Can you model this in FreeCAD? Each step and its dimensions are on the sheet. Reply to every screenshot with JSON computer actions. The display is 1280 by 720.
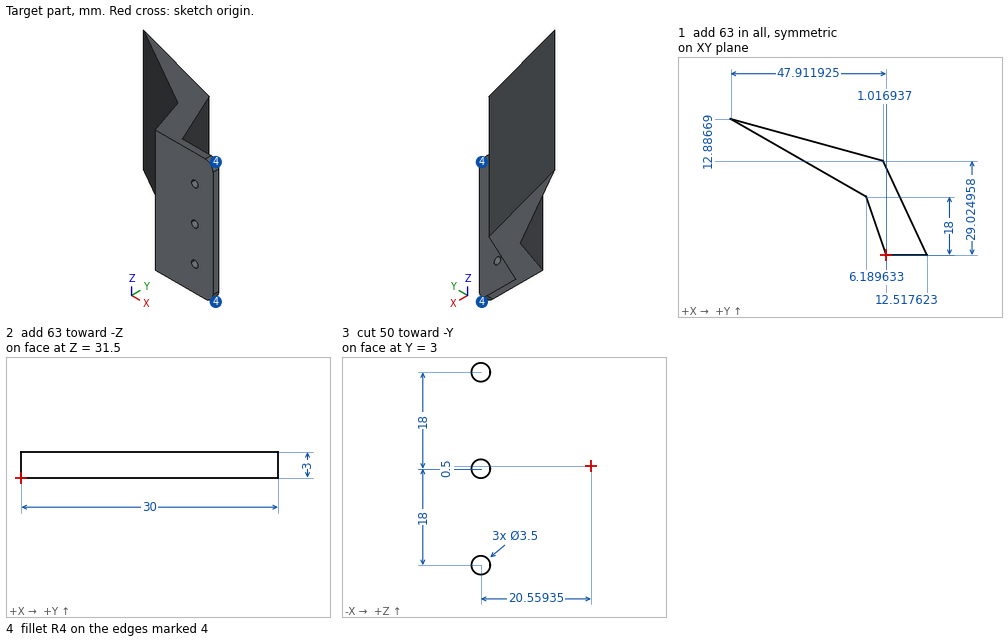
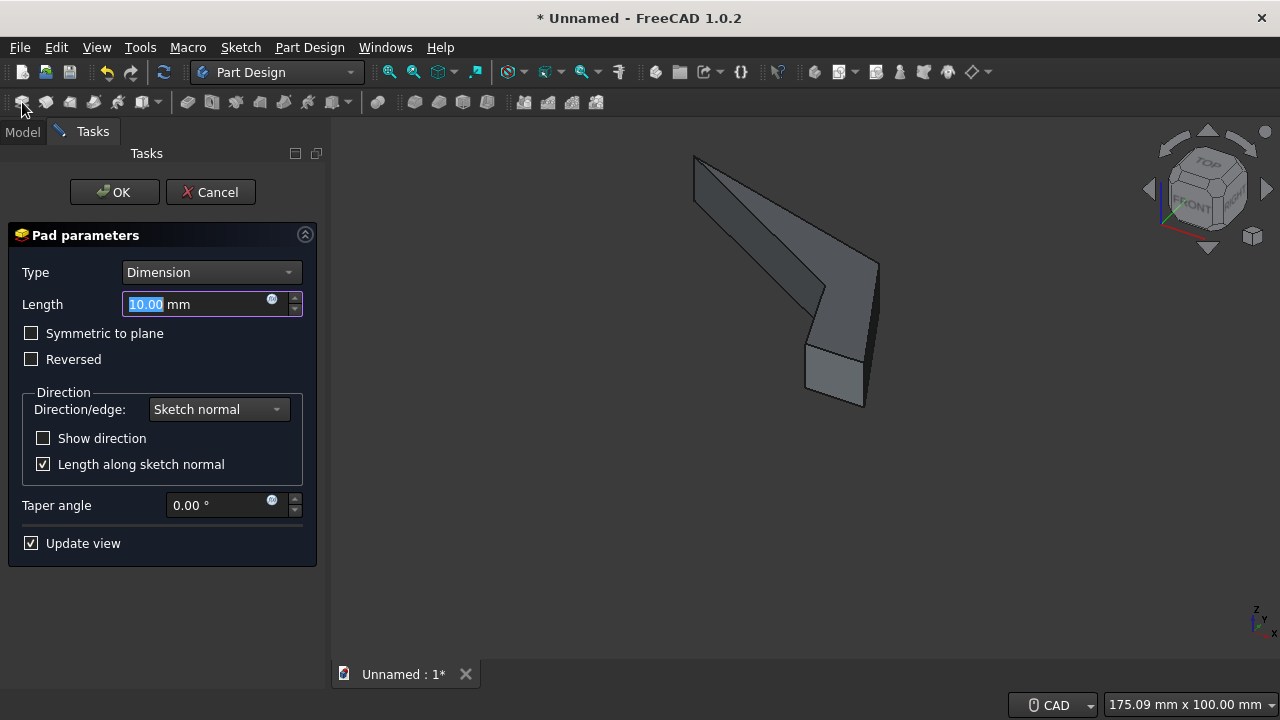
{"action": "type", "text": "63"}
{"action": "key", "text": "Tab"}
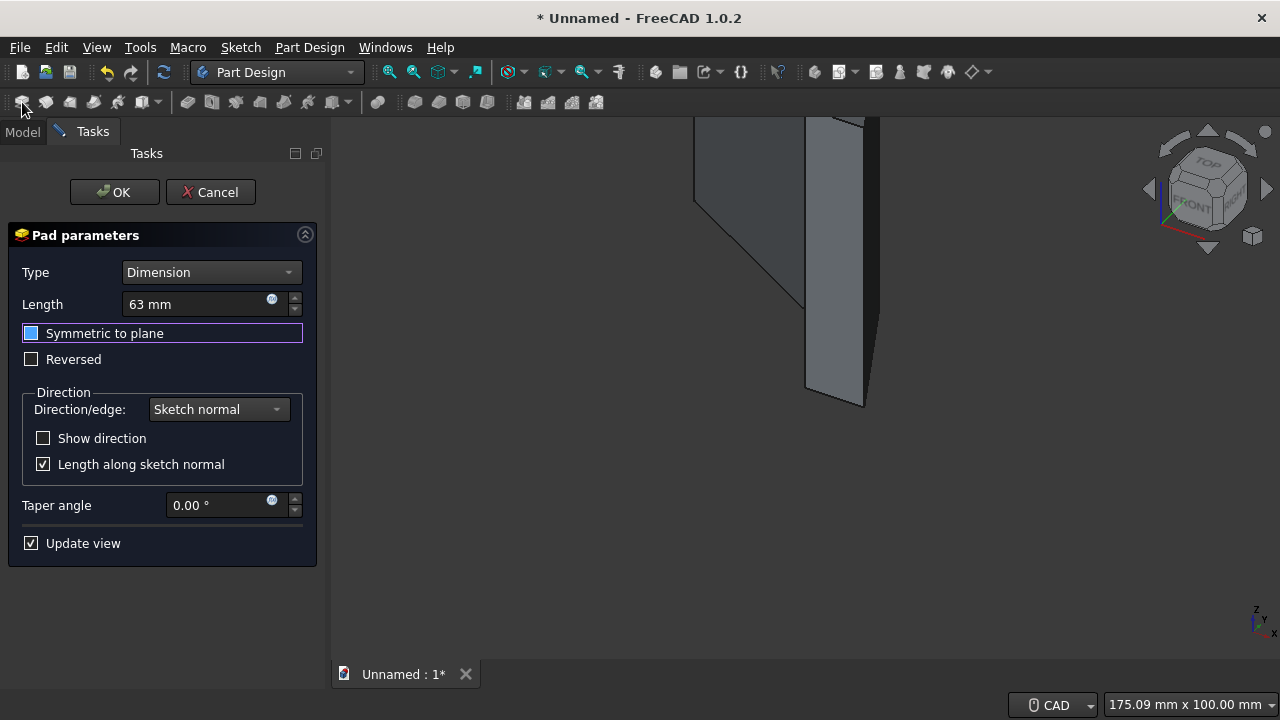
{"action": "left_click", "coordinate": [30, 333]}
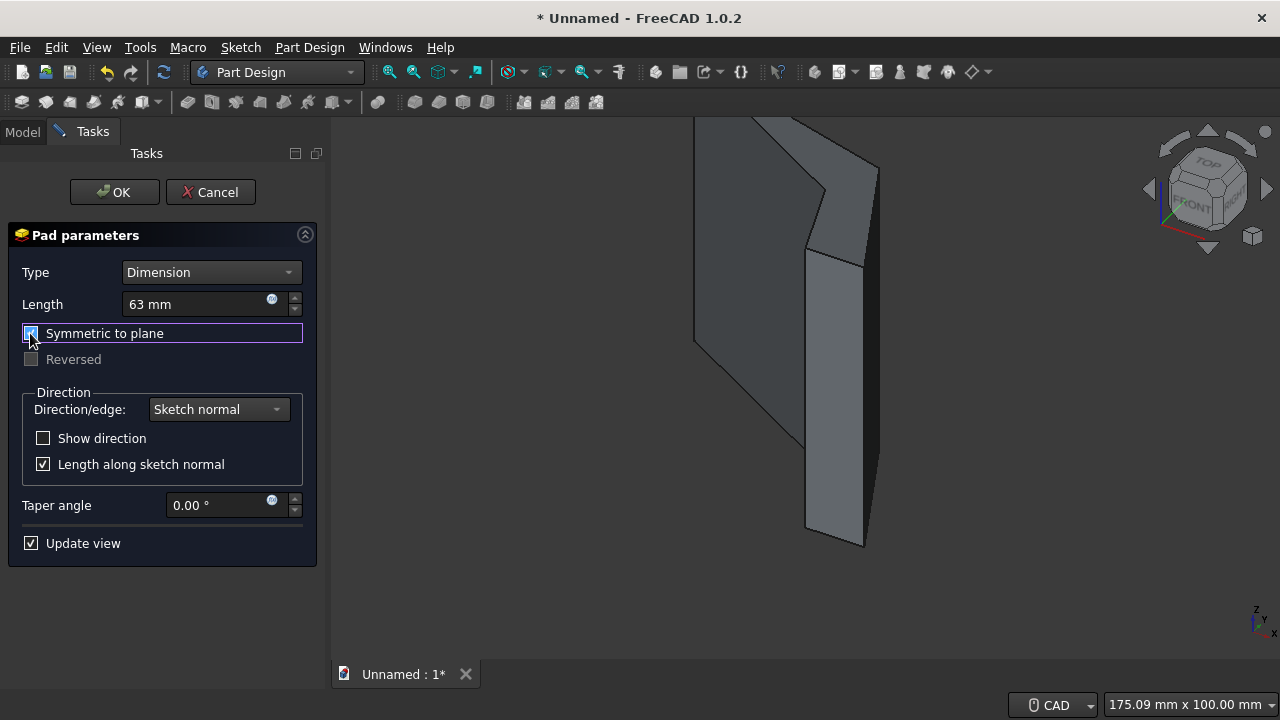
{"action": "left_click", "coordinate": [115, 192]}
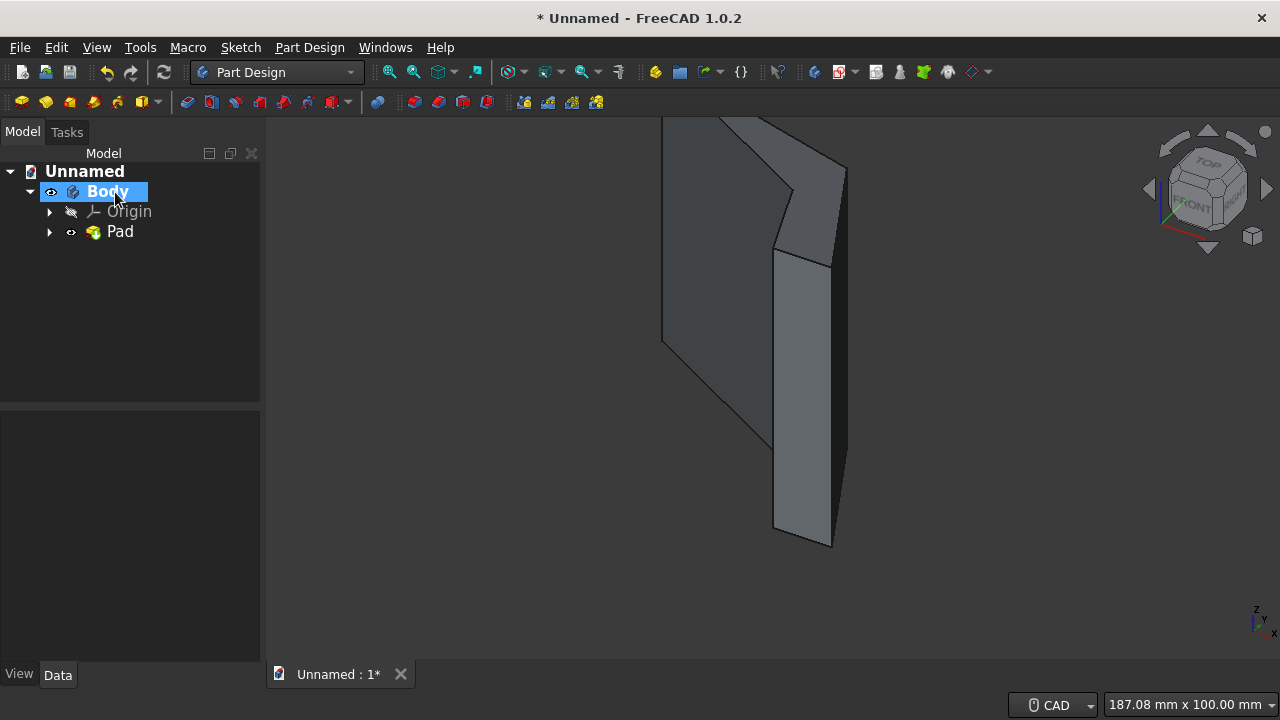
{"action": "key", "text": "v f"}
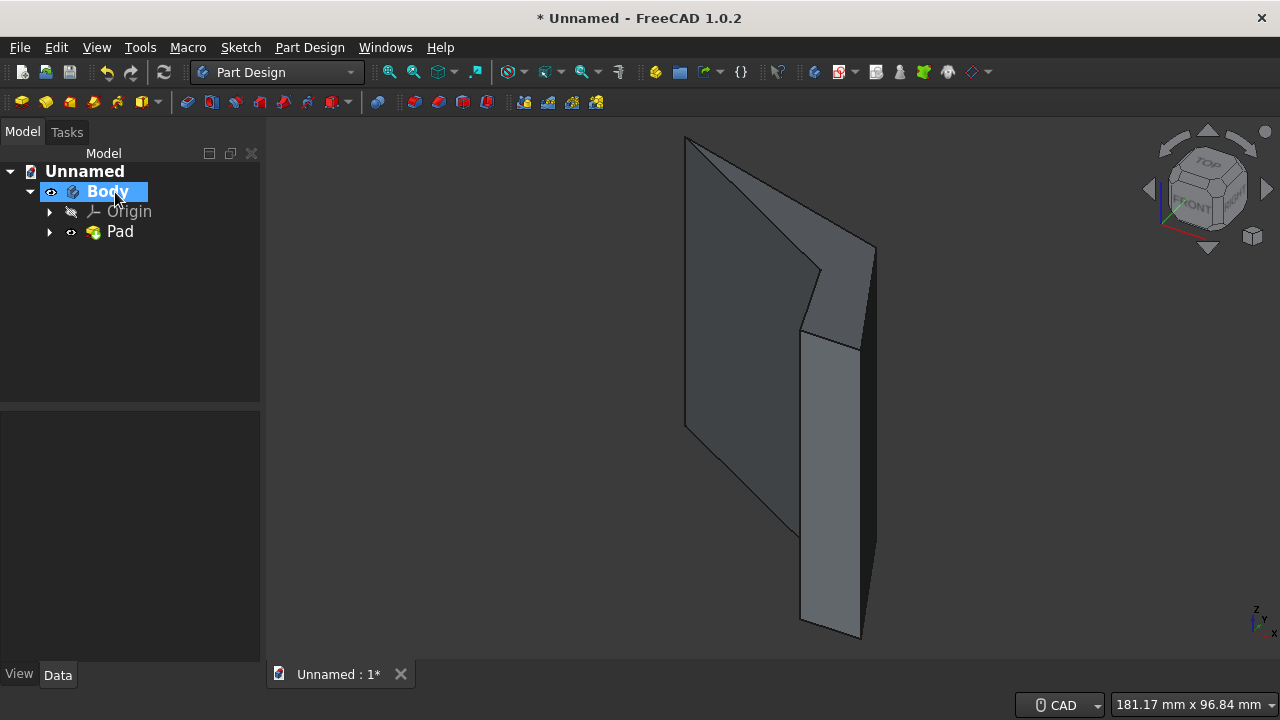
{"action": "left_click", "coordinate": [840, 287]}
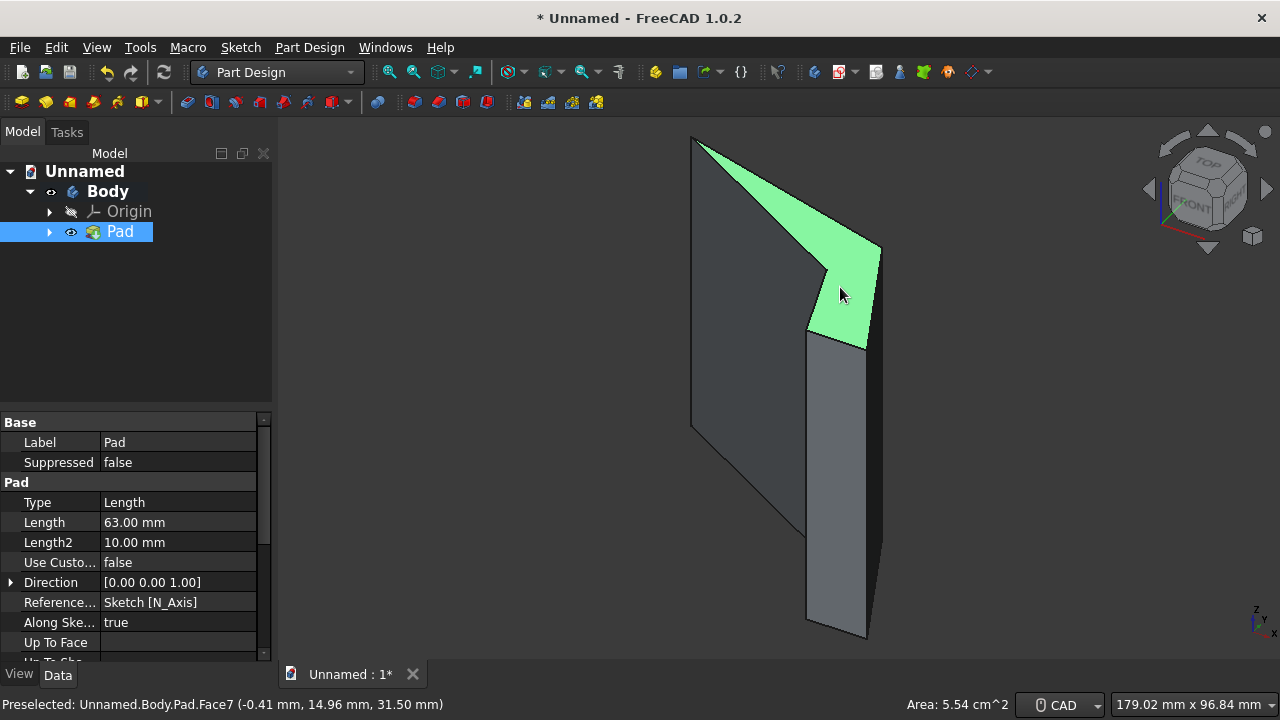
{"action": "left_click", "coordinate": [840, 72]}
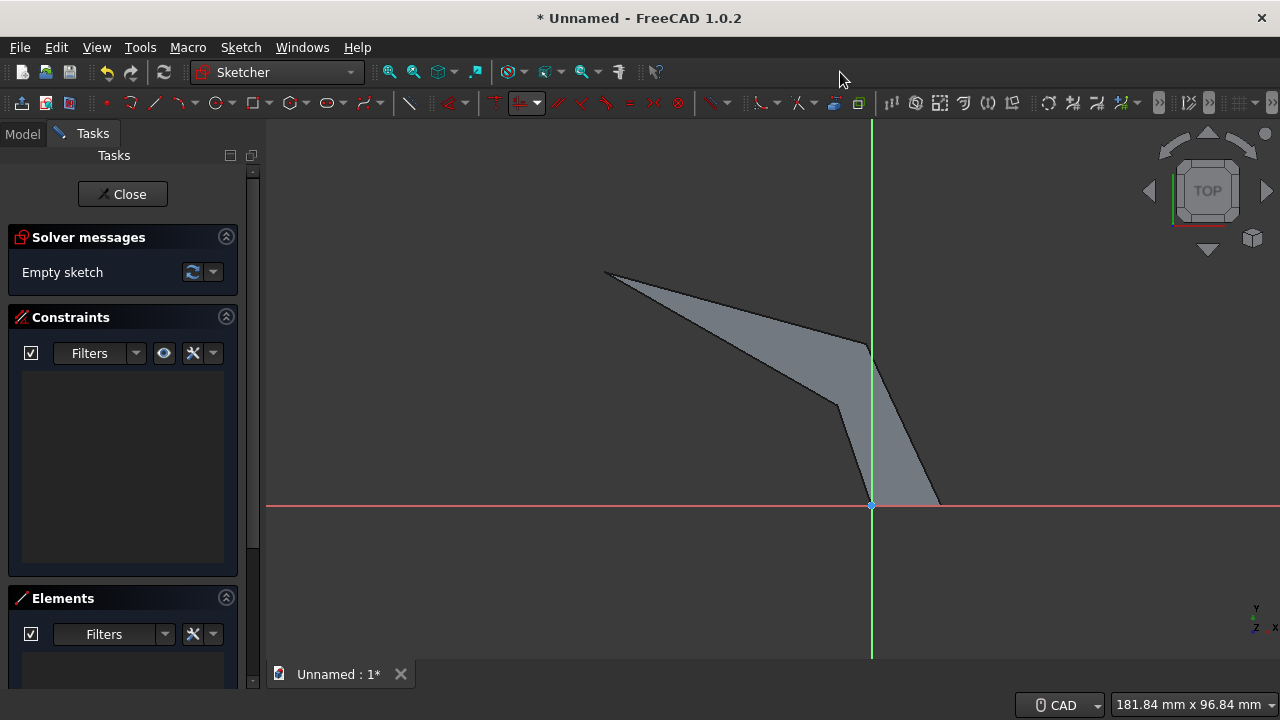
{"action": "scroll", "coordinate": [1063, 544], "scroll_direction": "up", "scroll_amount": 6}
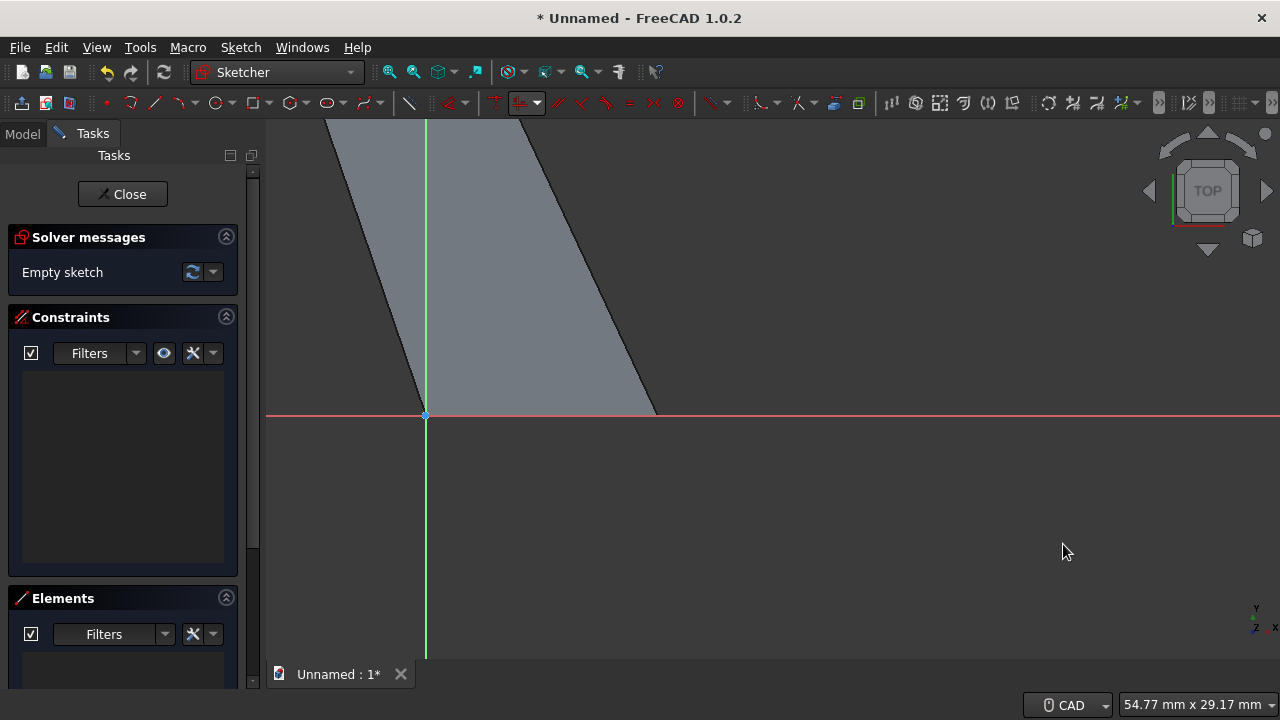
{"action": "left_click", "coordinate": [254, 104]}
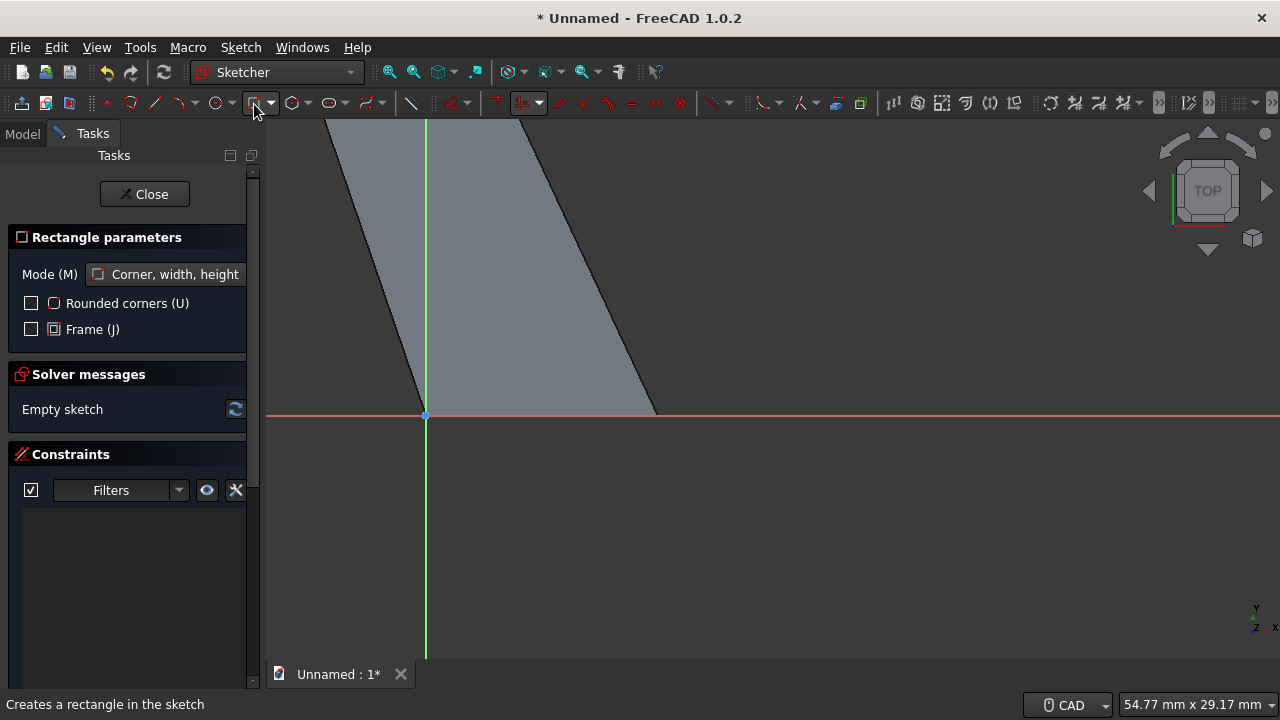
{"action": "left_click", "coordinate": [426, 416]}
{"action": "mouse_move", "coordinate": [981, 360]}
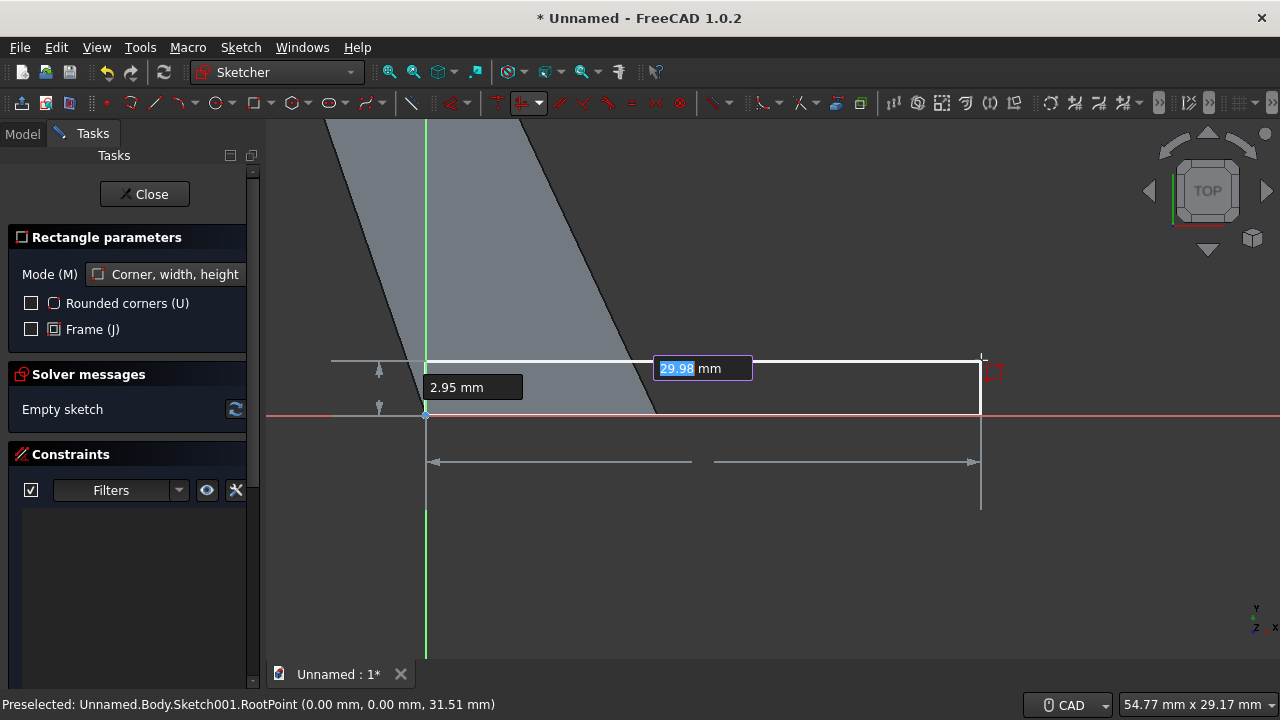
{"action": "type", "text": "30"}
{"action": "key", "text": "Tab"}
{"action": "type", "text": "3"}
{"action": "key", "text": "Return"}
{"action": "key", "text": "Escape"}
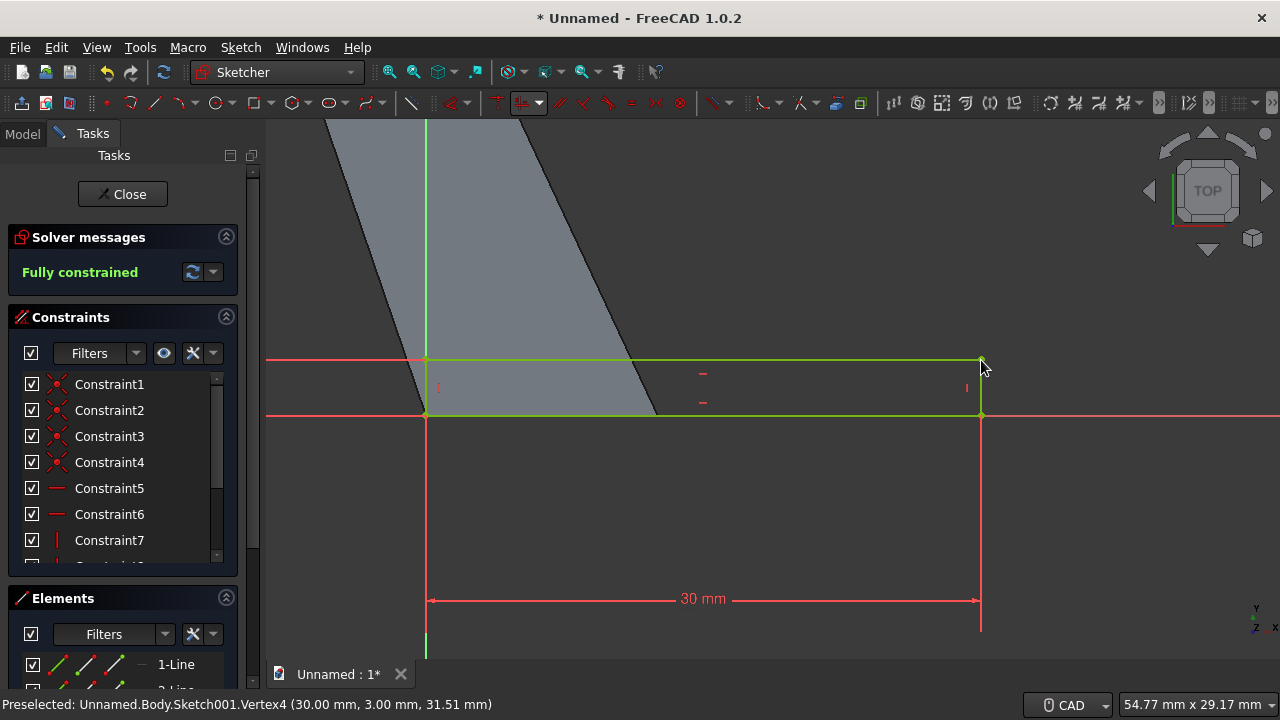
{"action": "left_click", "coordinate": [123, 194]}